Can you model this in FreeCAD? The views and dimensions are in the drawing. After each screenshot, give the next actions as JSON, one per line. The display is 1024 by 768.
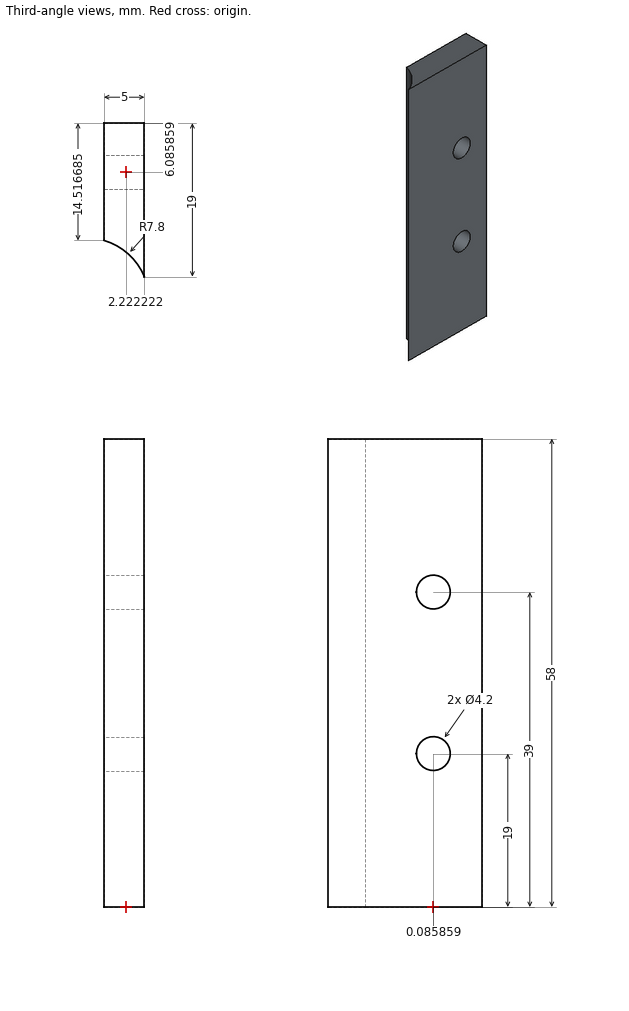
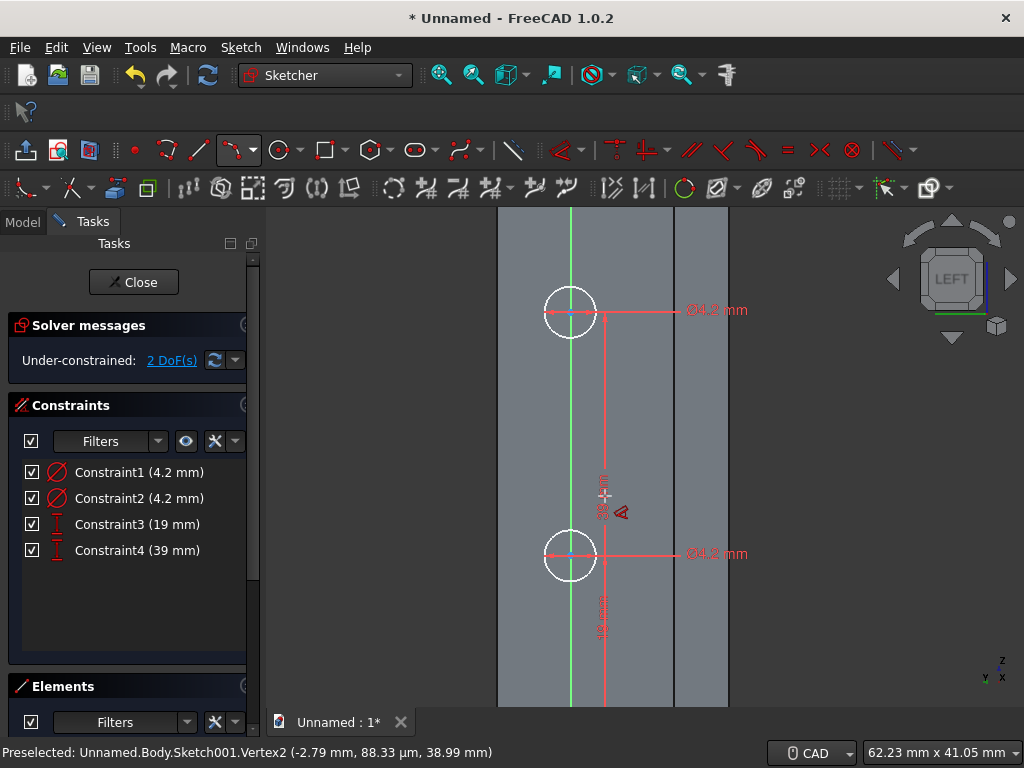
{"action": "scroll", "coordinate": [570, 556], "scroll_direction": "up", "scroll_amount": 19}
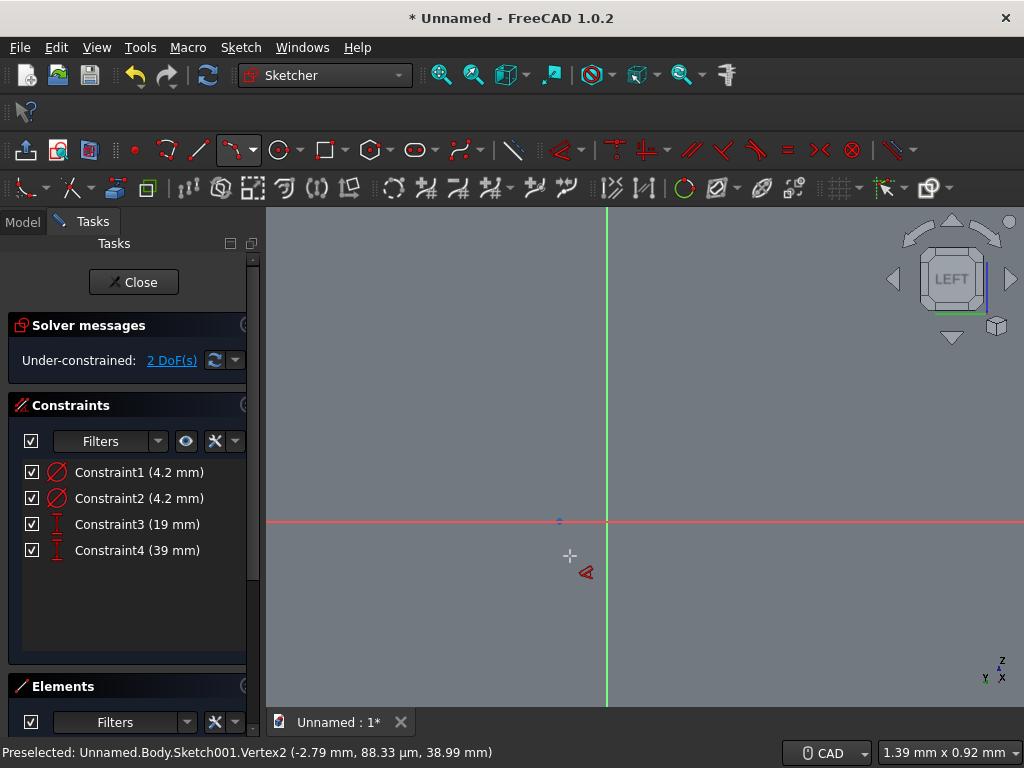
{"action": "left_click", "coordinate": [560, 522]}
{"action": "left_click", "coordinate": [583, 488]}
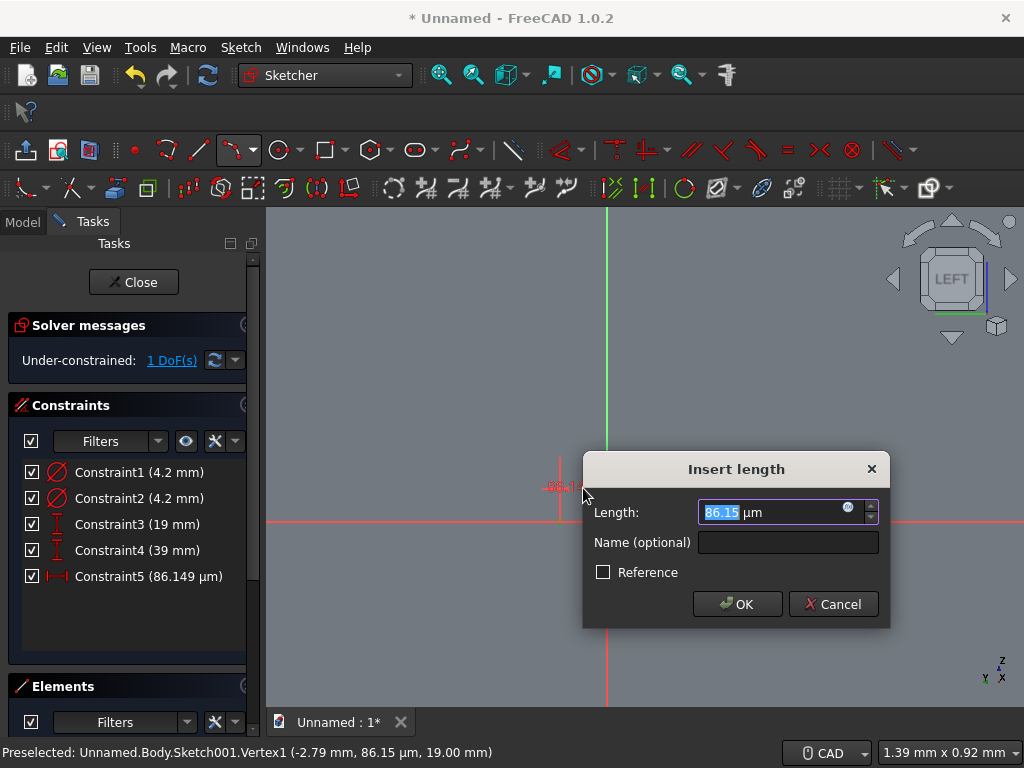
{"action": "key", "text": "ctrl+a"}
{"action": "type", "text": "0.085859 mm"}
{"action": "key", "text": "Return"}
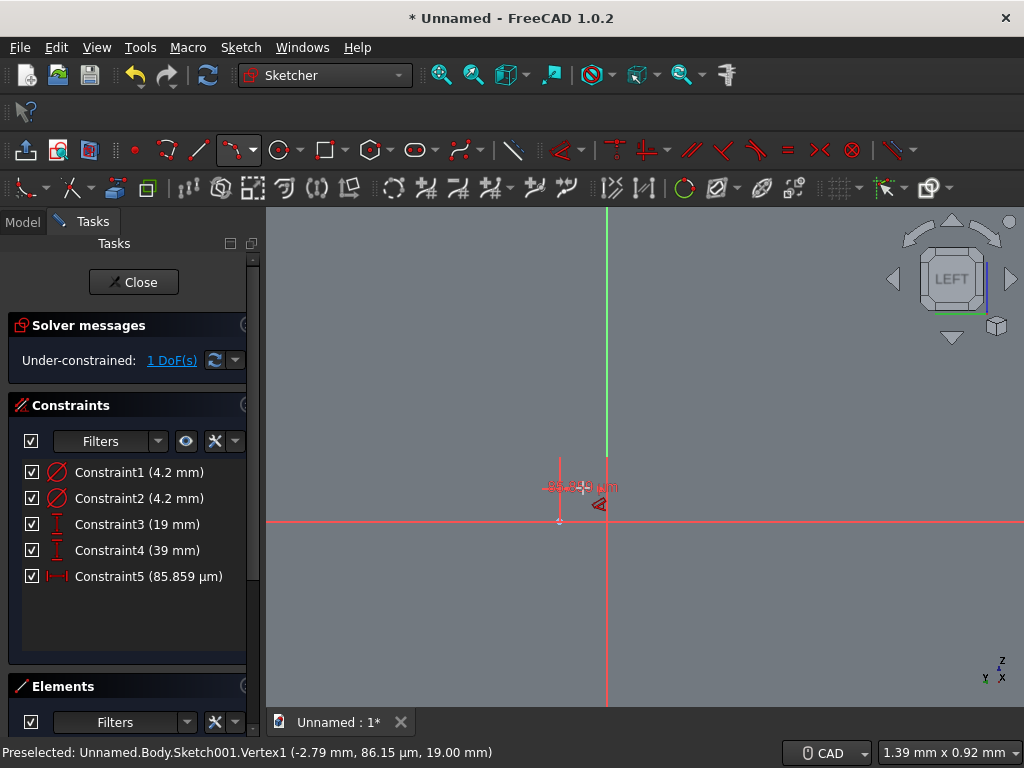
{"action": "scroll", "coordinate": [576, 457], "scroll_direction": "down", "scroll_amount": 15}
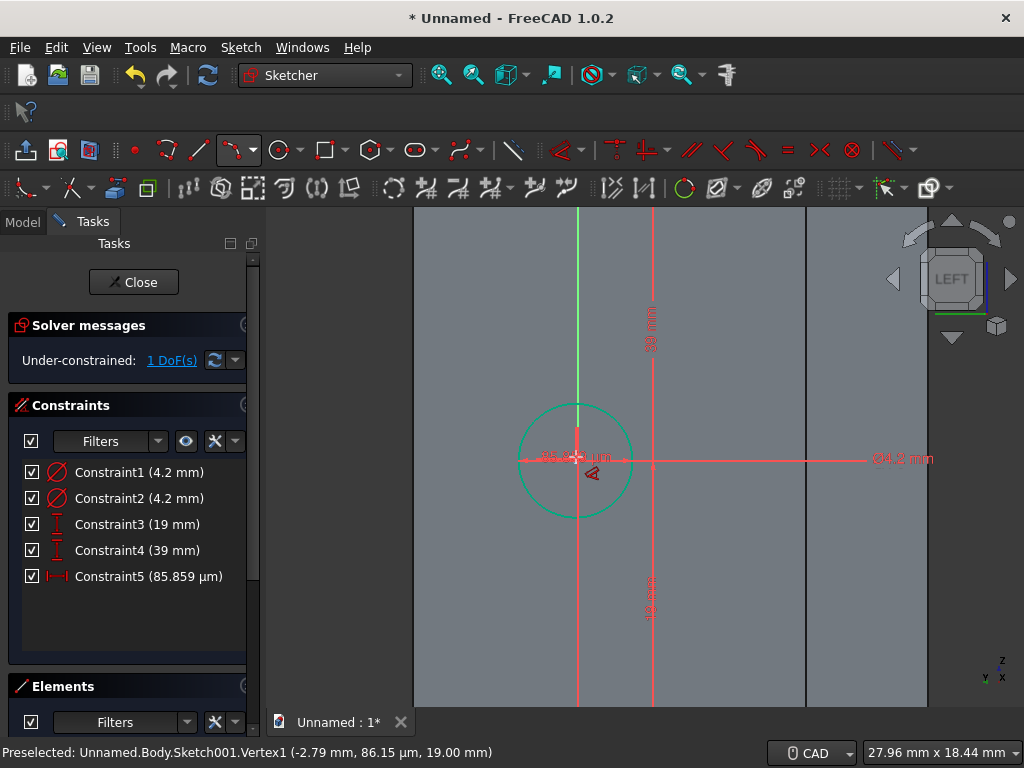
{"action": "scroll", "coordinate": [577, 474], "scroll_direction": "down", "scroll_amount": 6}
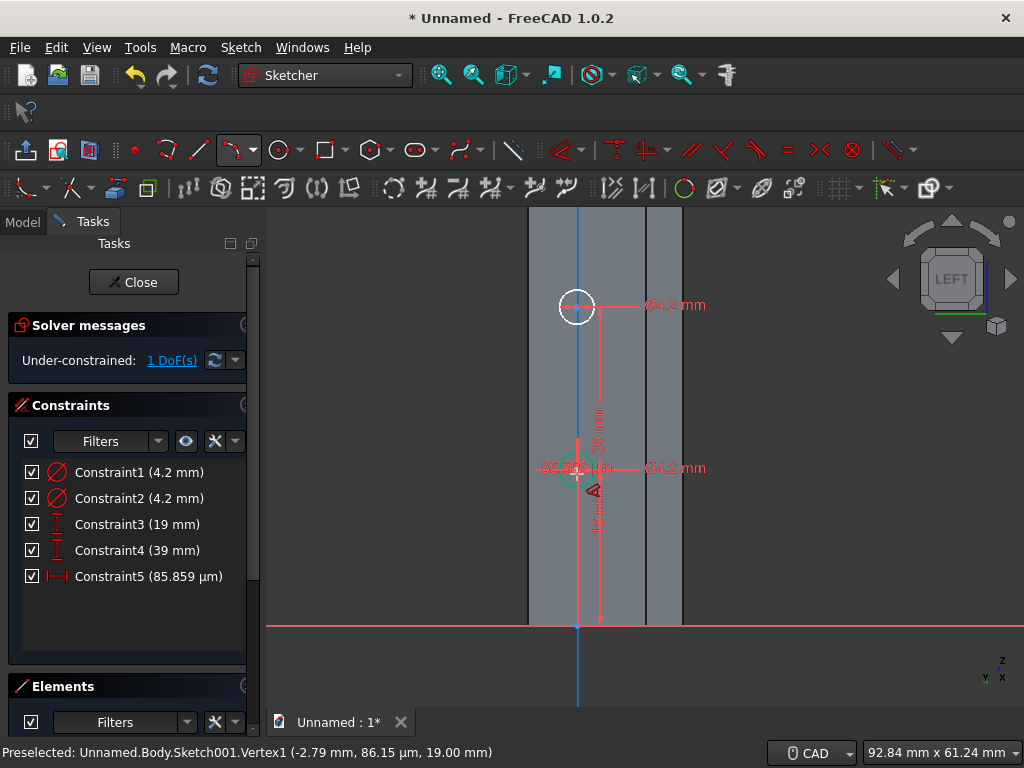
{"action": "scroll", "coordinate": [577, 307], "scroll_direction": "up", "scroll_amount": 21}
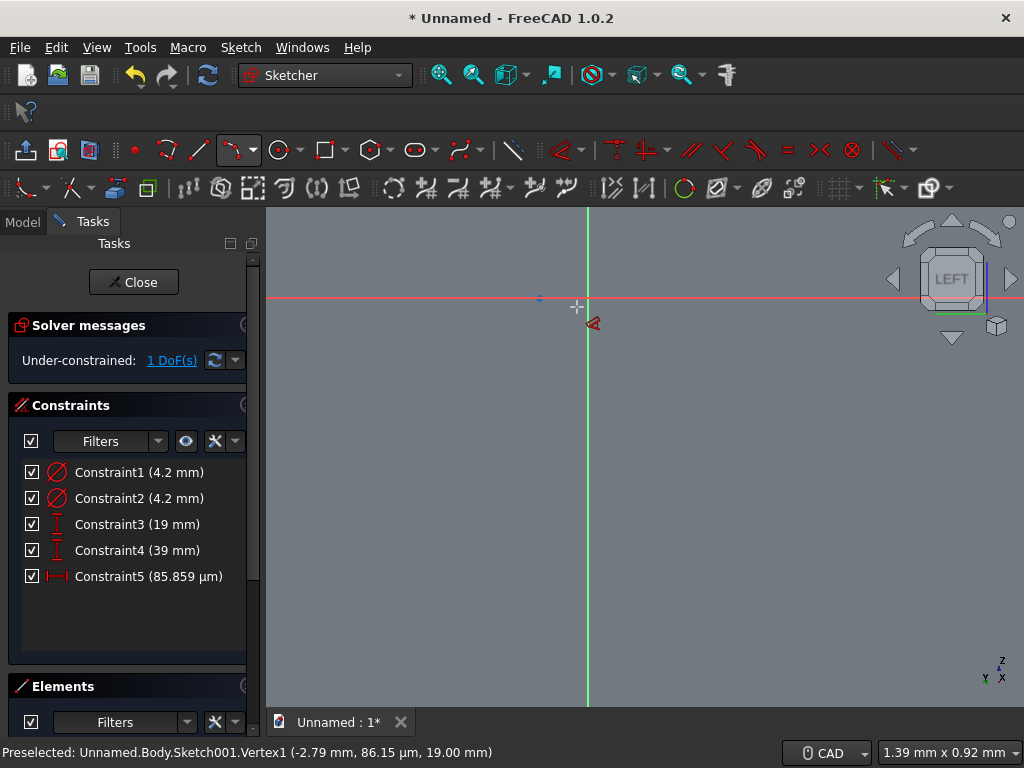
{"action": "left_click", "coordinate": [540, 298]}
{"action": "left_click", "coordinate": [564, 264]}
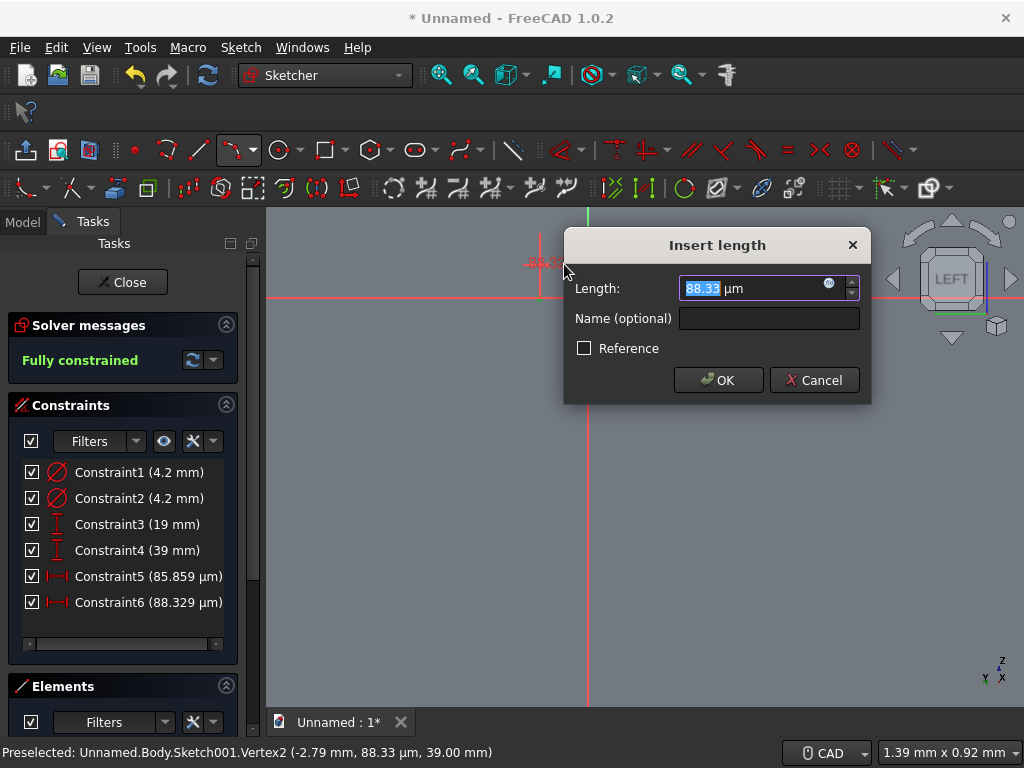
{"action": "key", "text": "ctrl+a"}
{"action": "type", "text": "0.085859 mm"}
{"action": "key", "text": "Return"}
{"action": "key", "text": "Escape"}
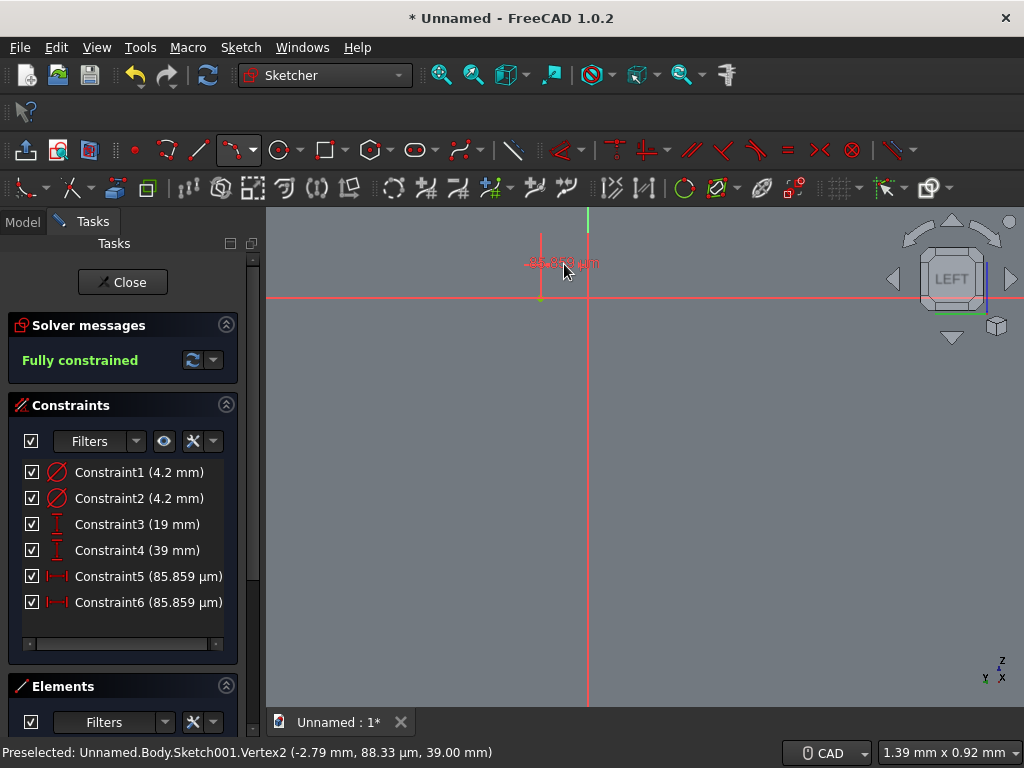
{"action": "left_click", "coordinate": [123, 282]}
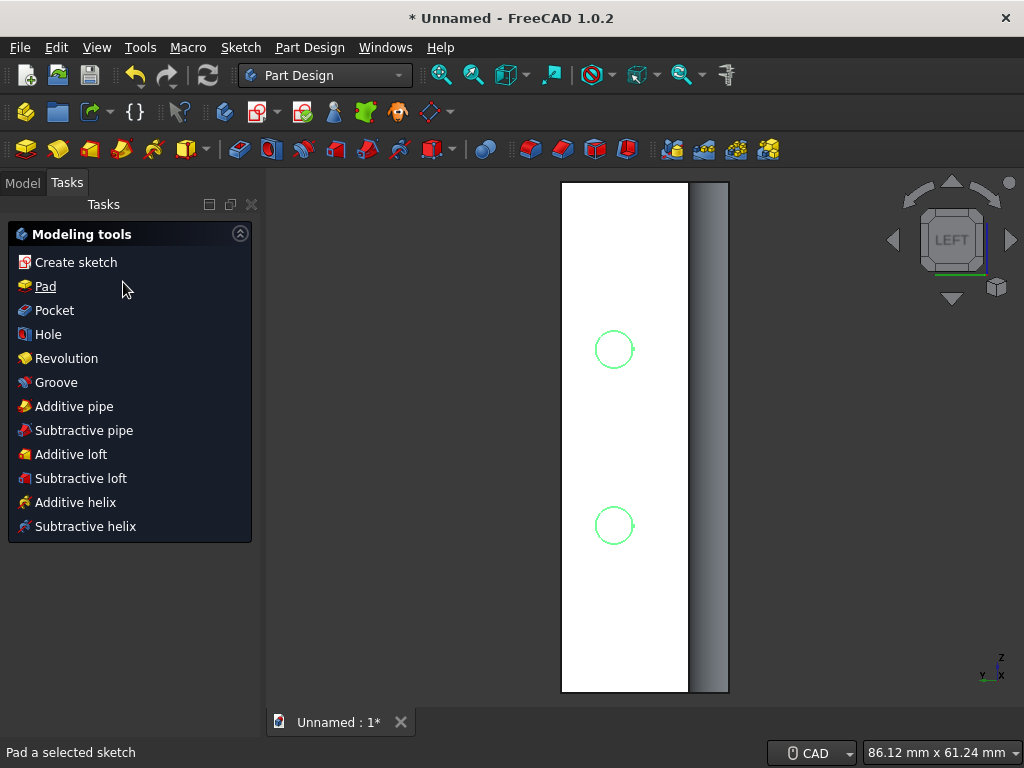
{"action": "left_click", "coordinate": [240, 150]}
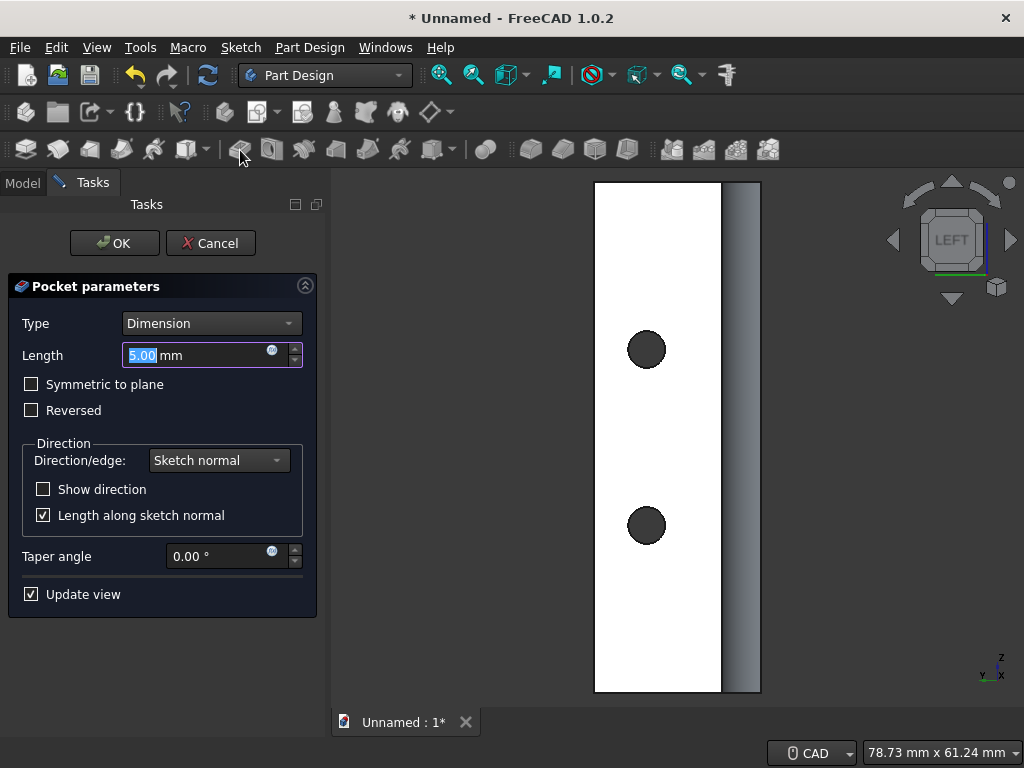
{"action": "left_click", "coordinate": [212, 324]}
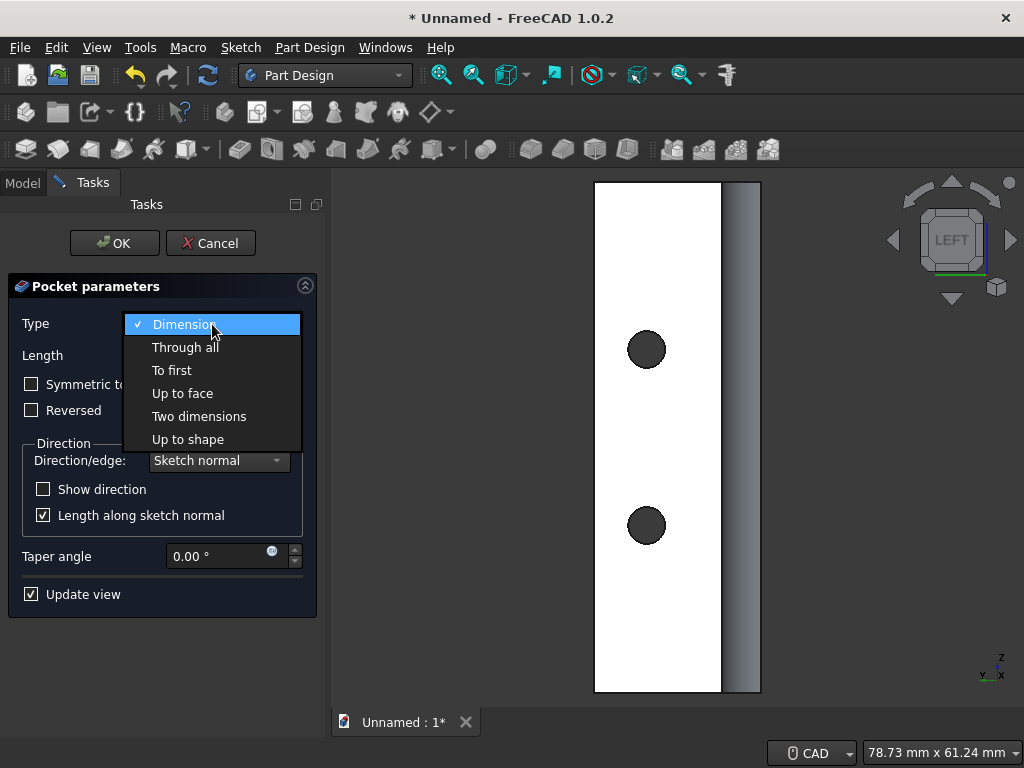
{"action": "left_click", "coordinate": [212, 348]}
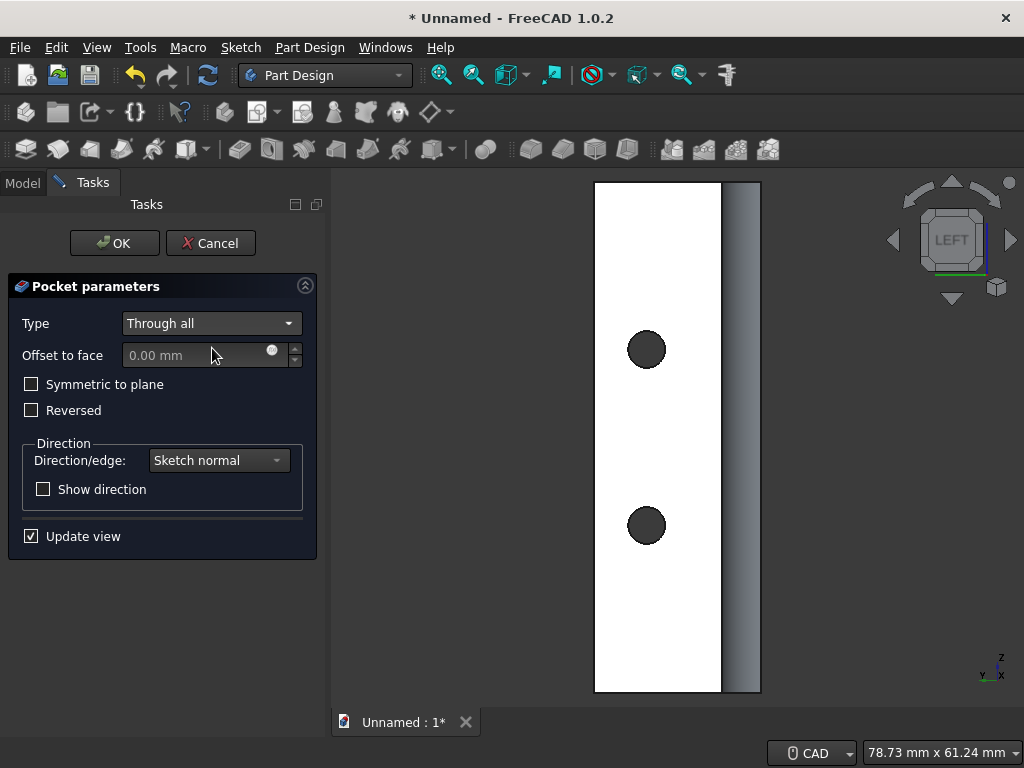
{"action": "left_click", "coordinate": [115, 243]}